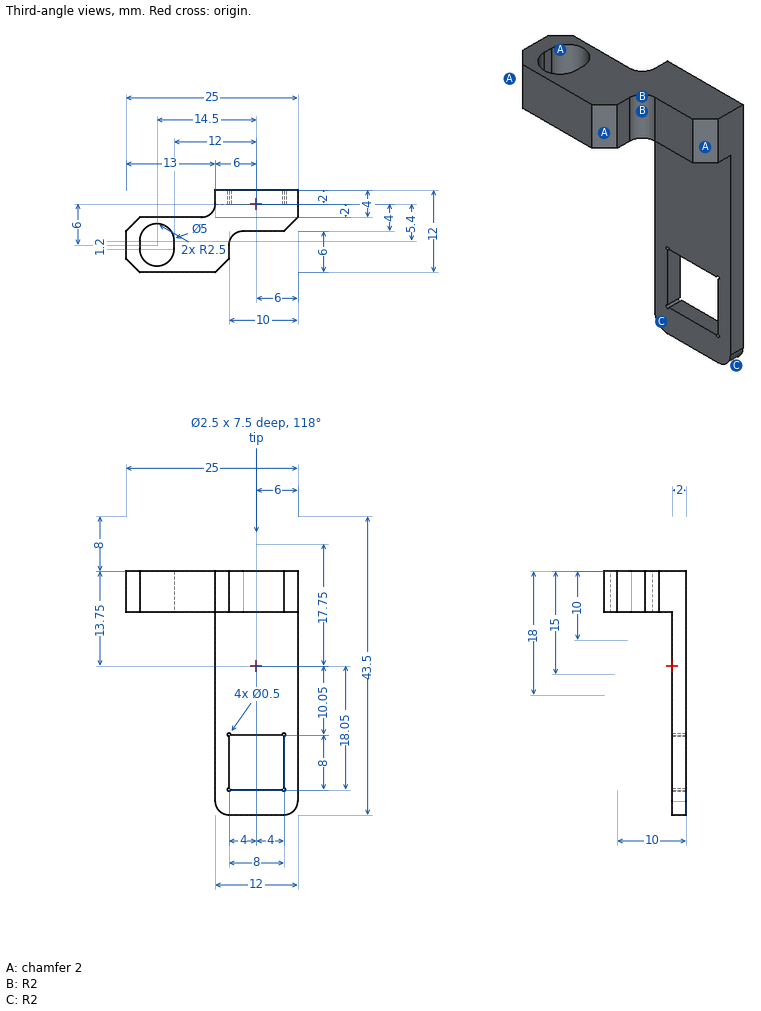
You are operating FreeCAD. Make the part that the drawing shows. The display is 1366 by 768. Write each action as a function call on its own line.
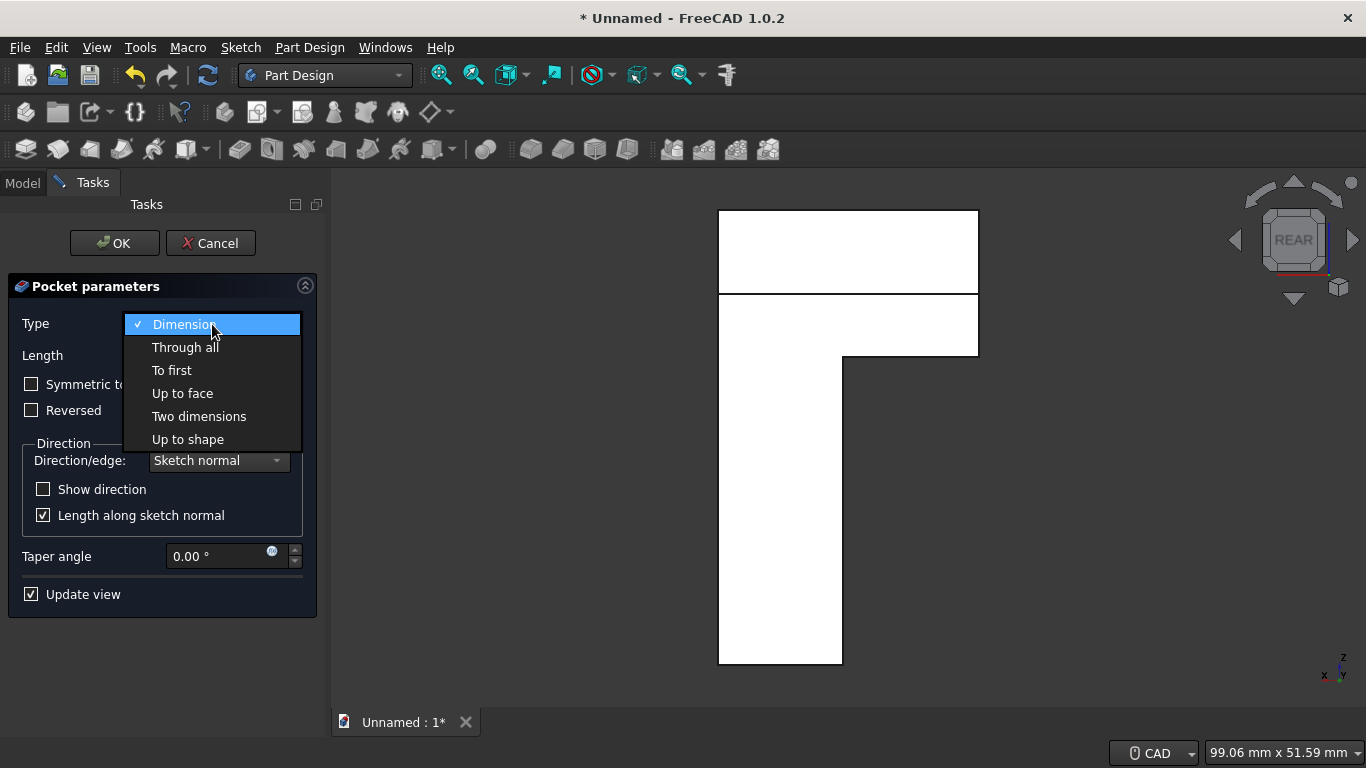
click(212, 348)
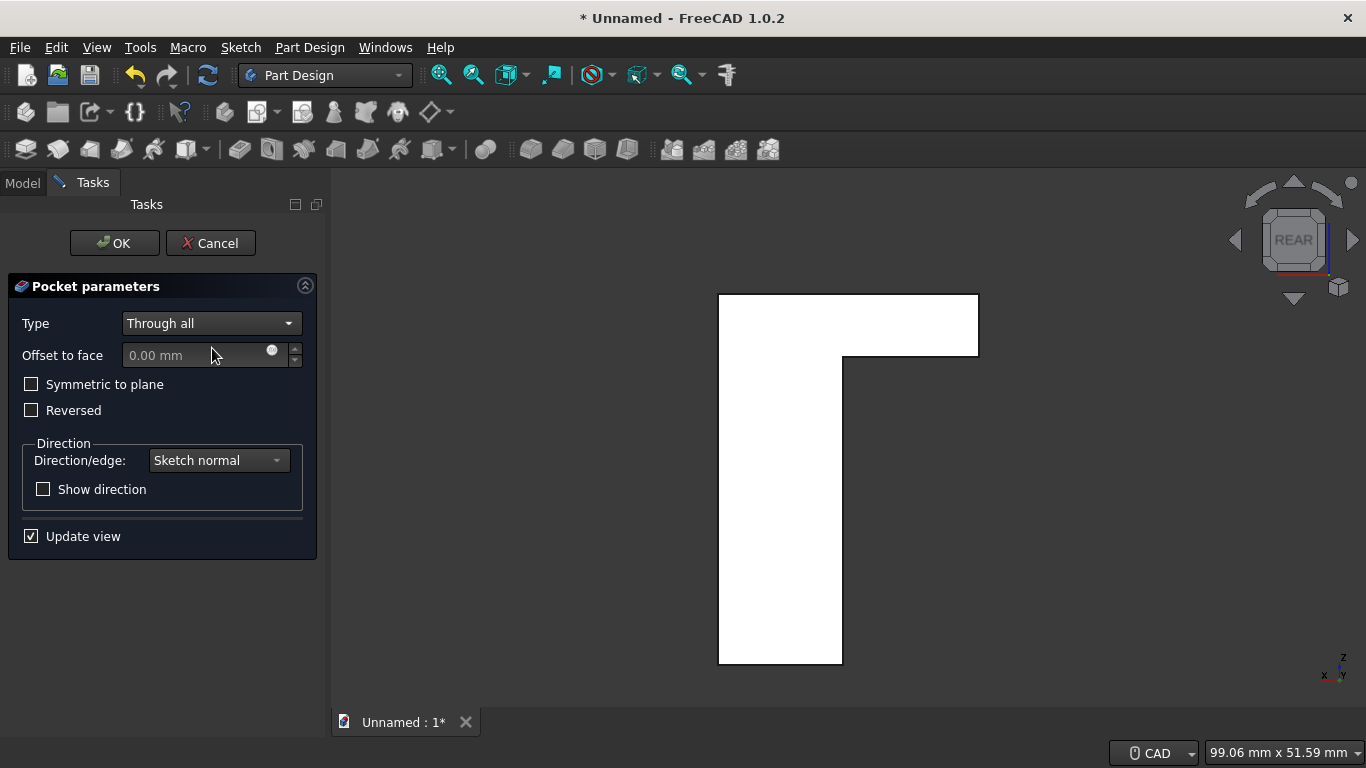
click(115, 243)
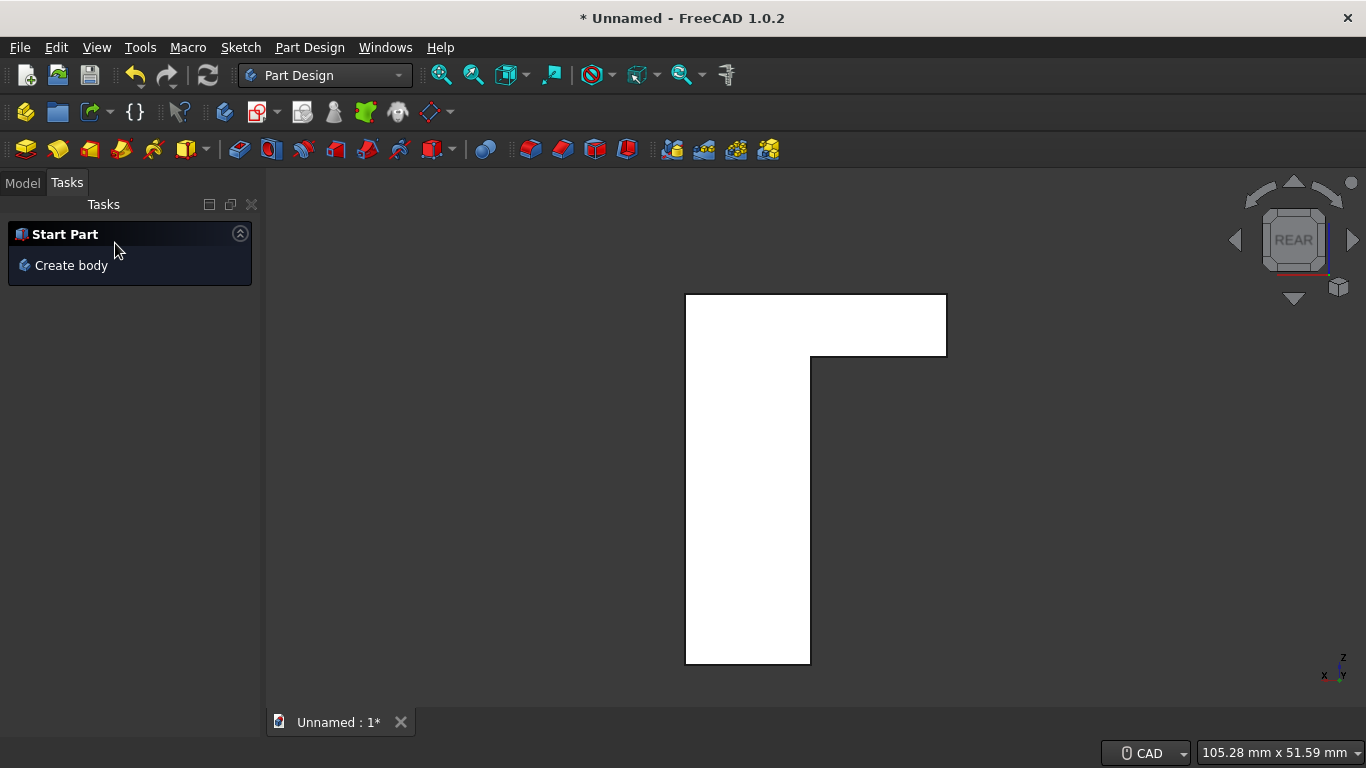
key(0)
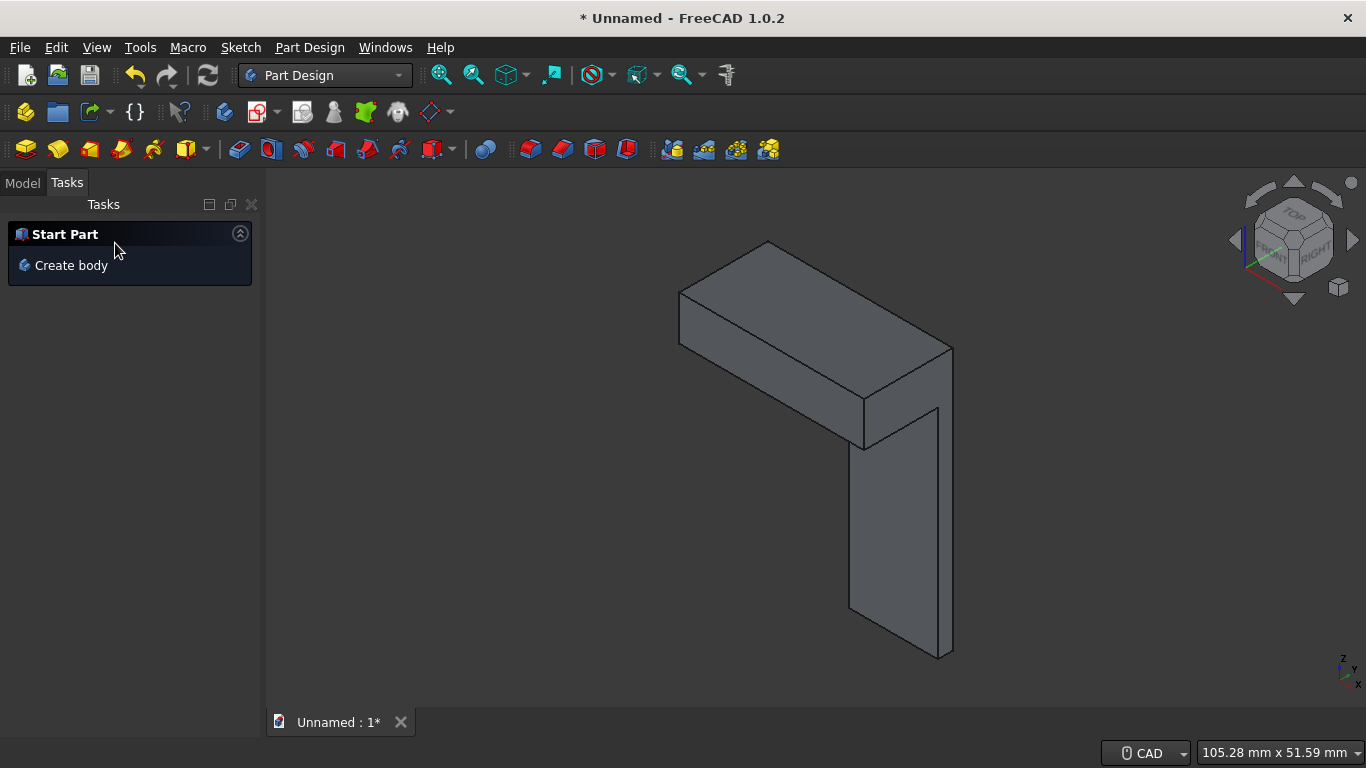
click(842, 334)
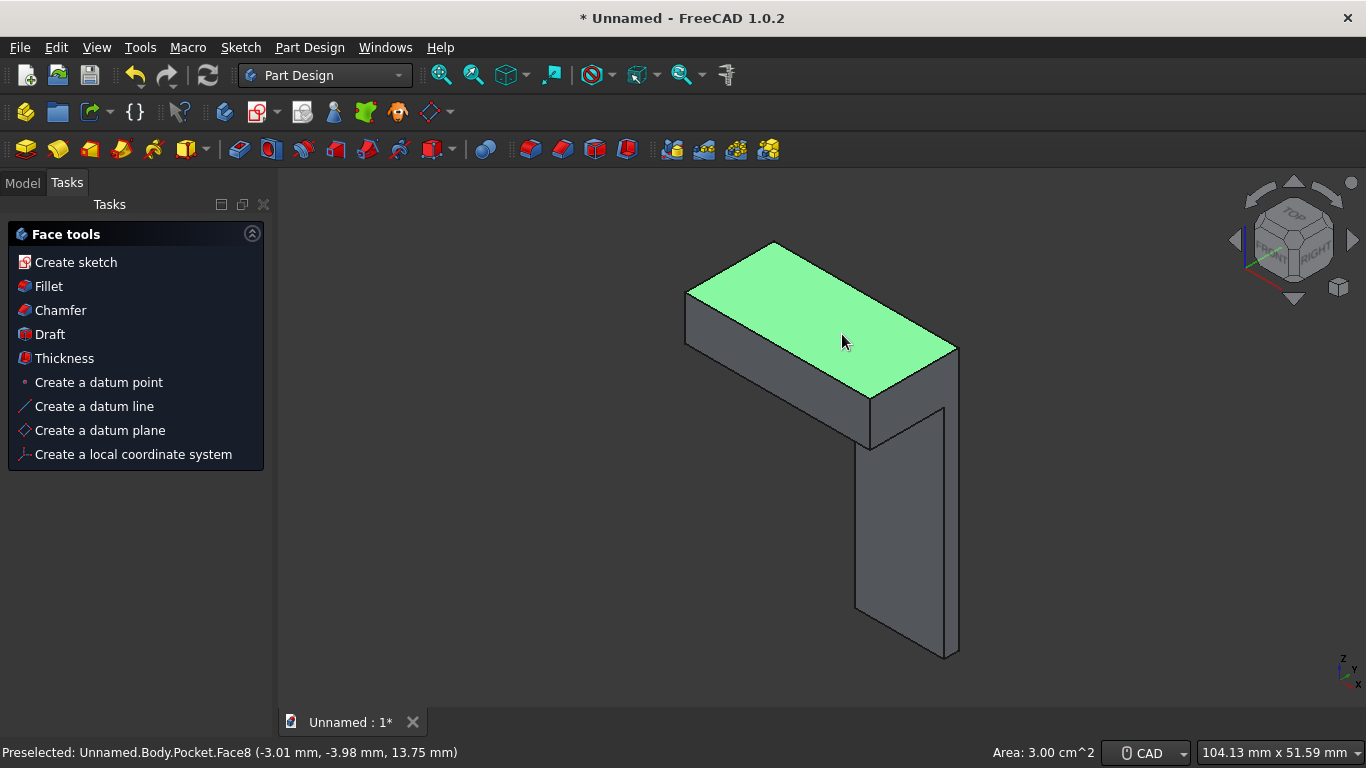
click(258, 112)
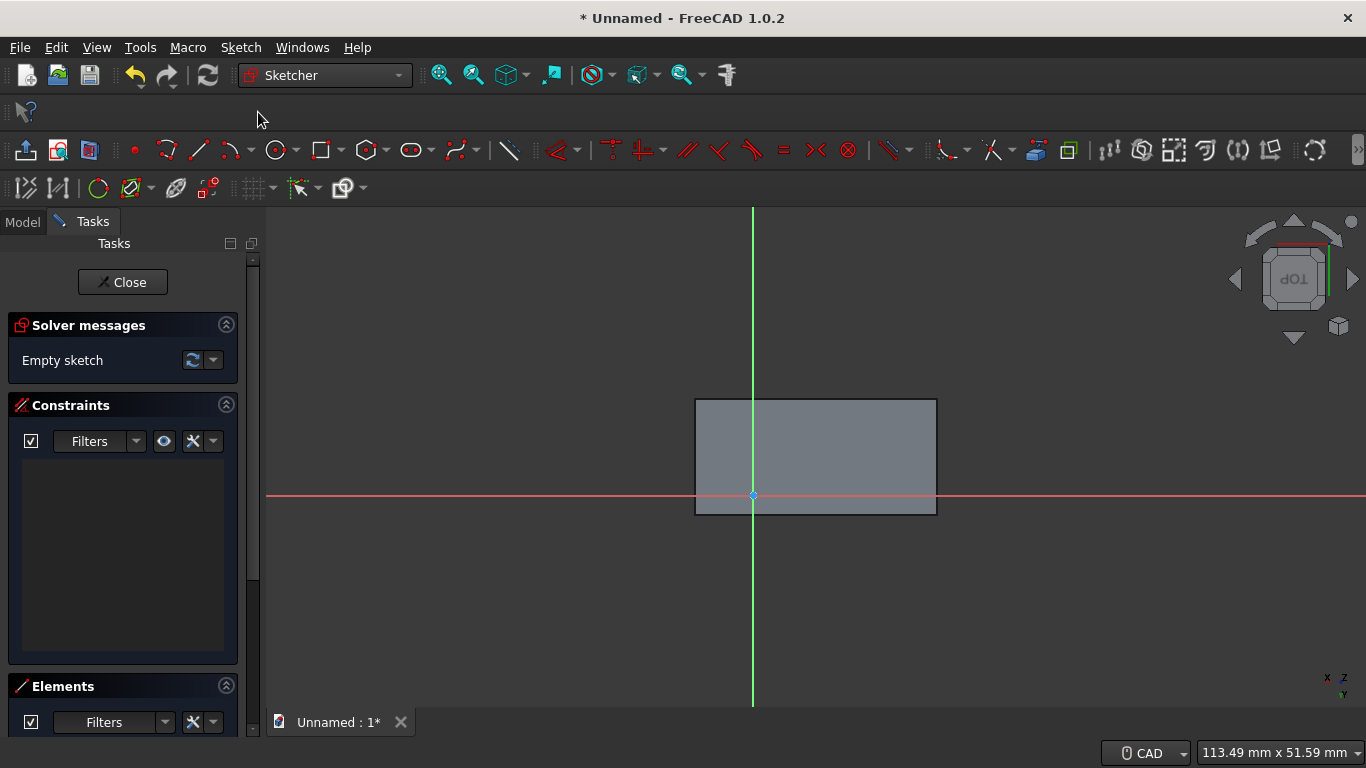
scroll(922, 434, up, 9)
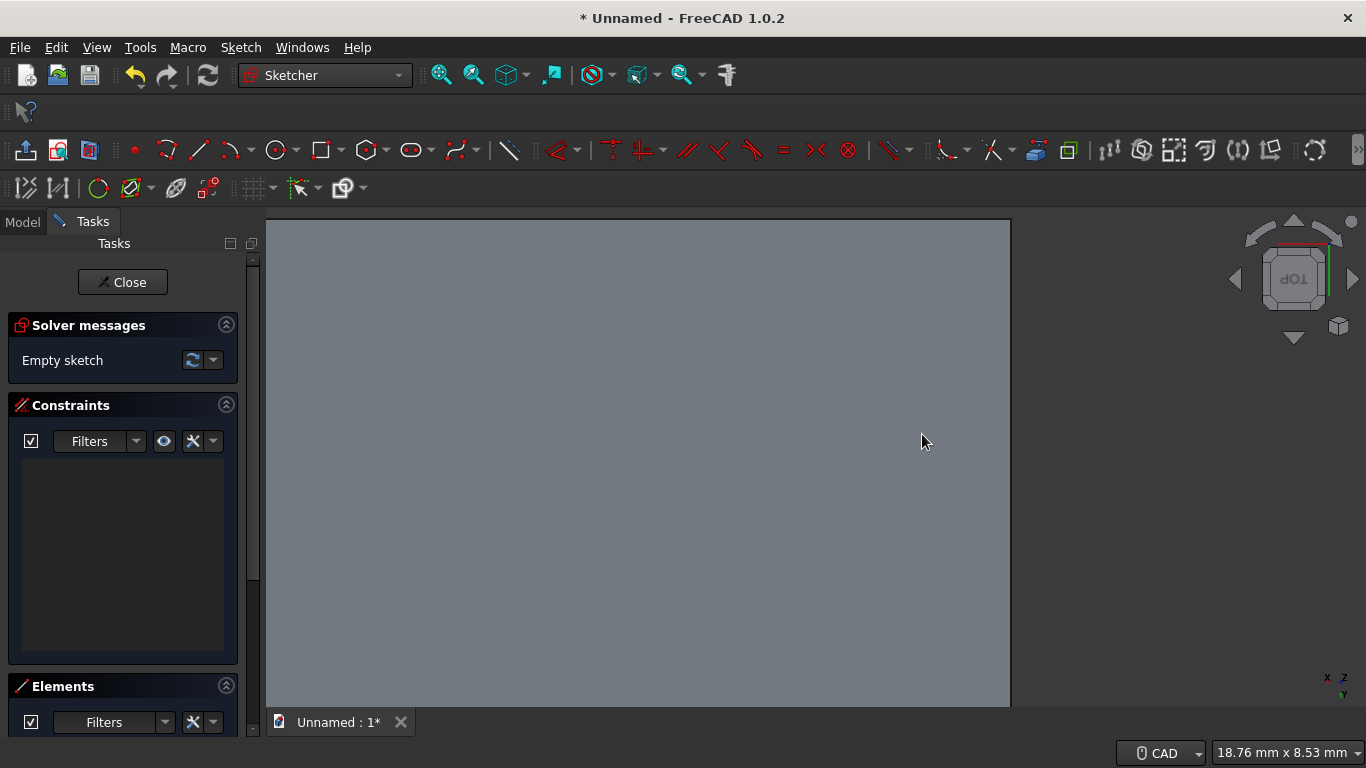
click(276, 150)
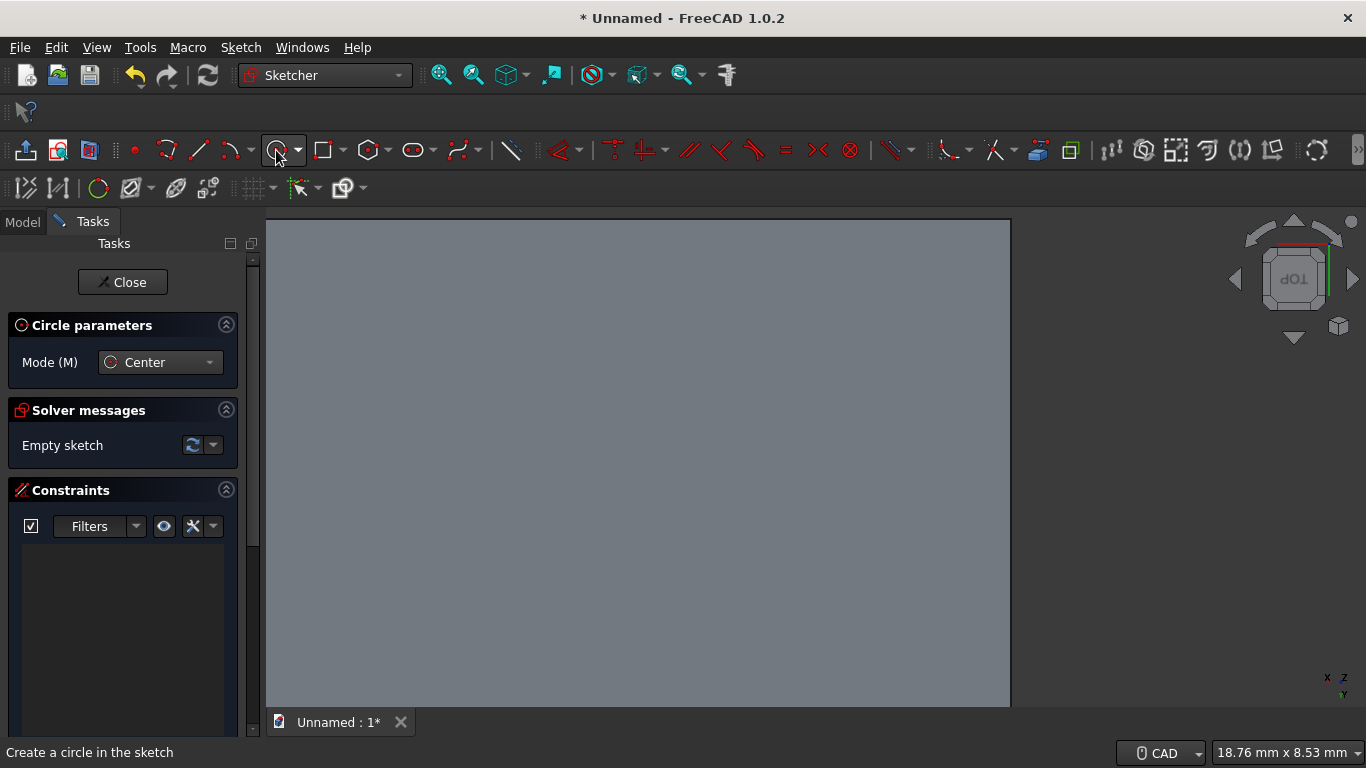
click(747, 454)
click(850, 350)
key(Escape)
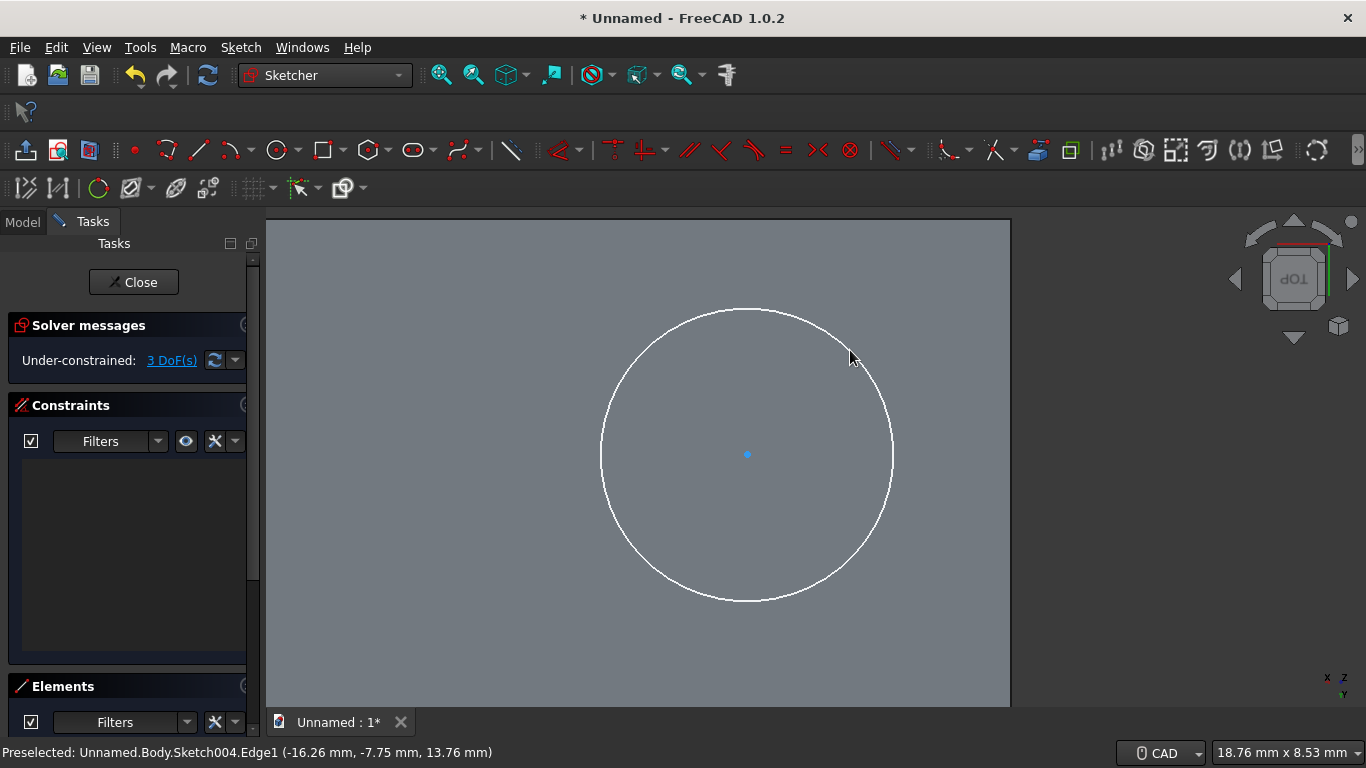
click(558, 150)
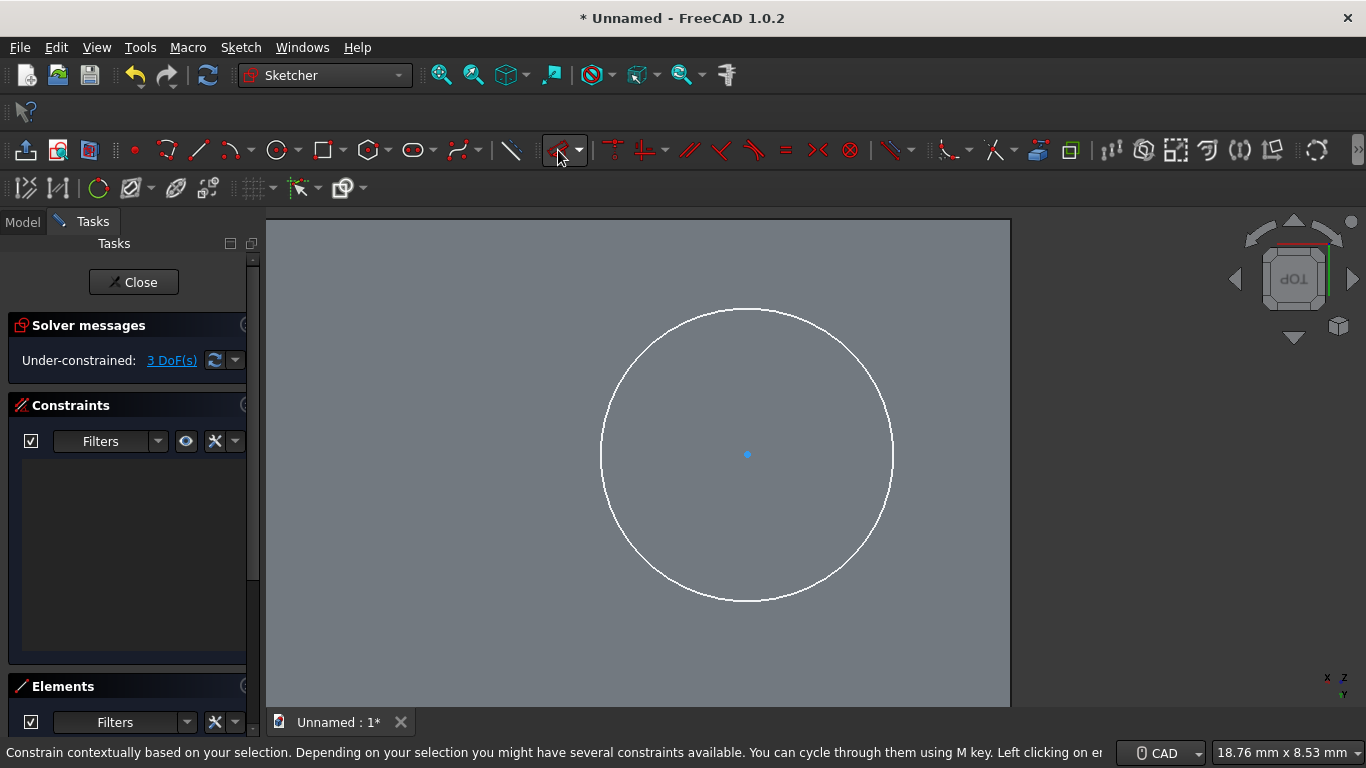
click(850, 351)
click(873, 328)